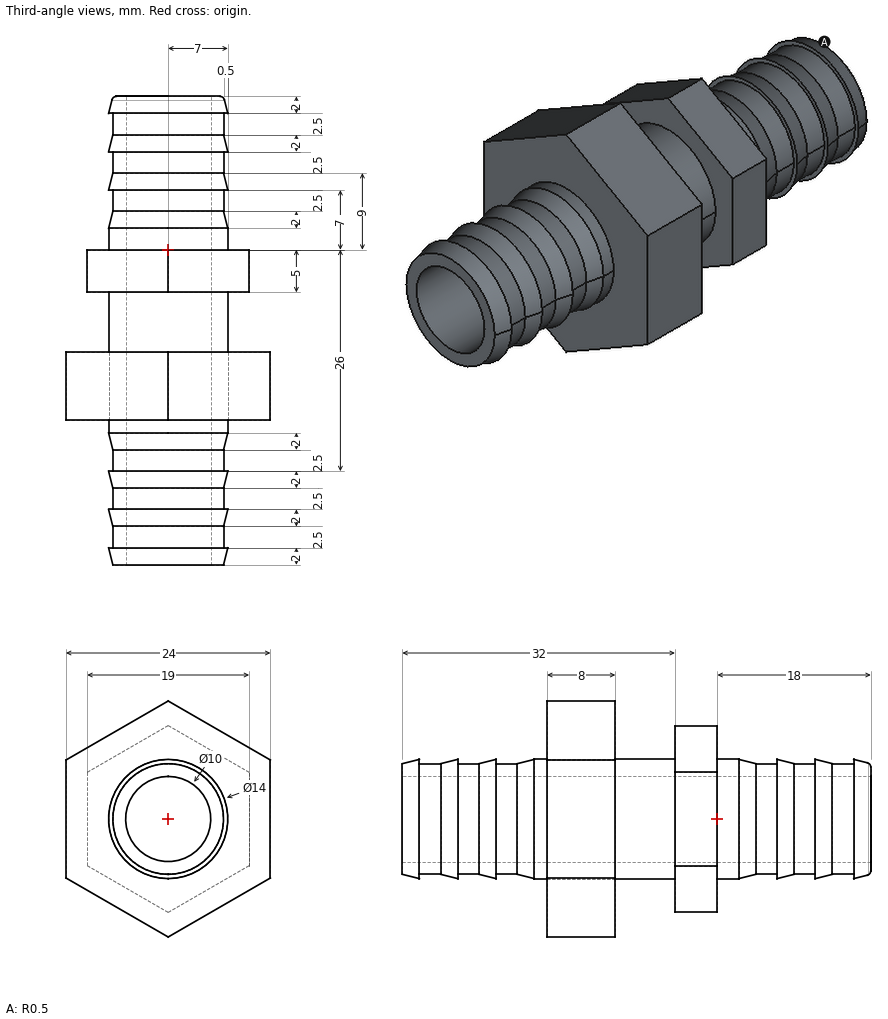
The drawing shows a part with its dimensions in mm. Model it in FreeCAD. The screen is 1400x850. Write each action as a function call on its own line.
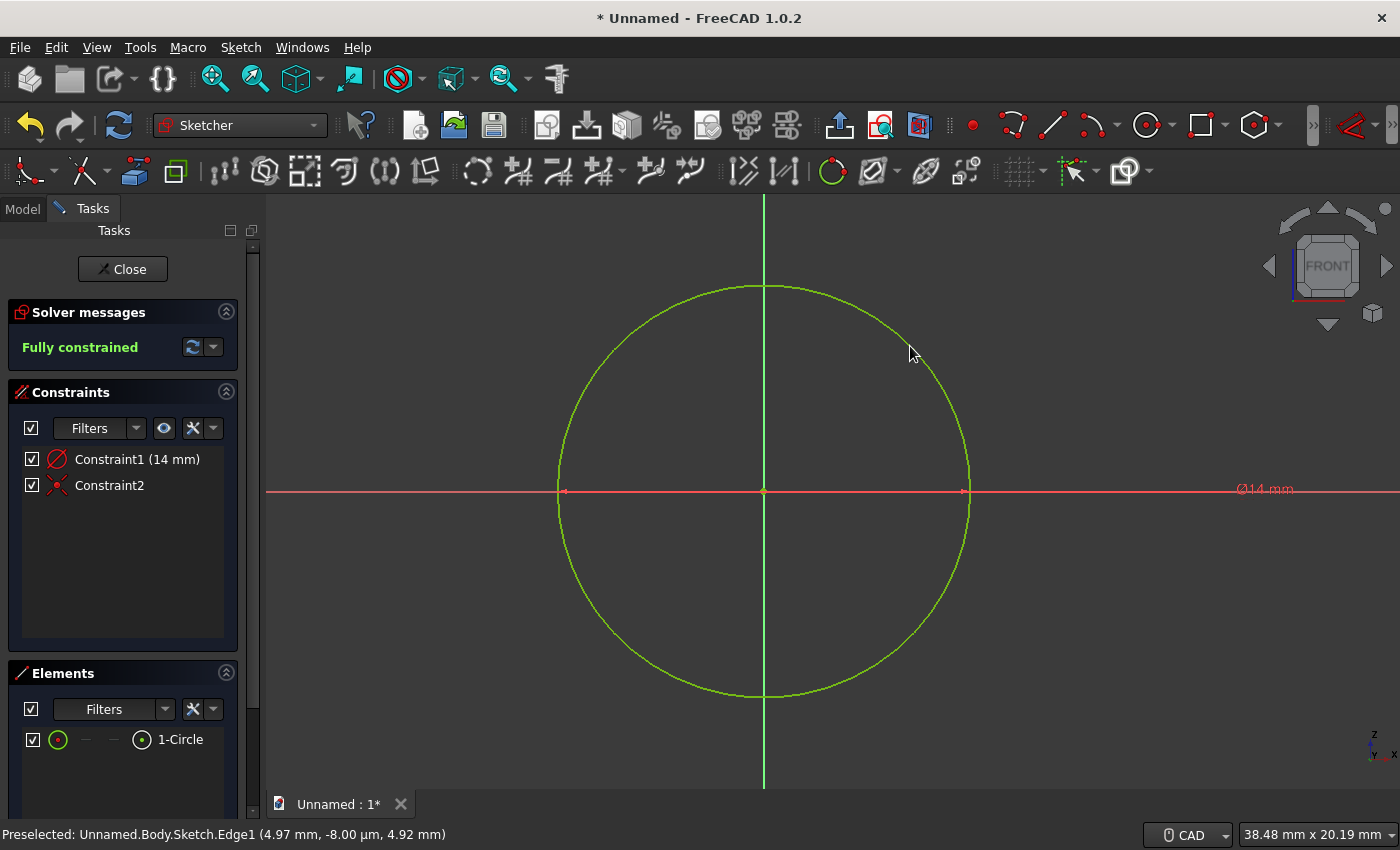
click(123, 269)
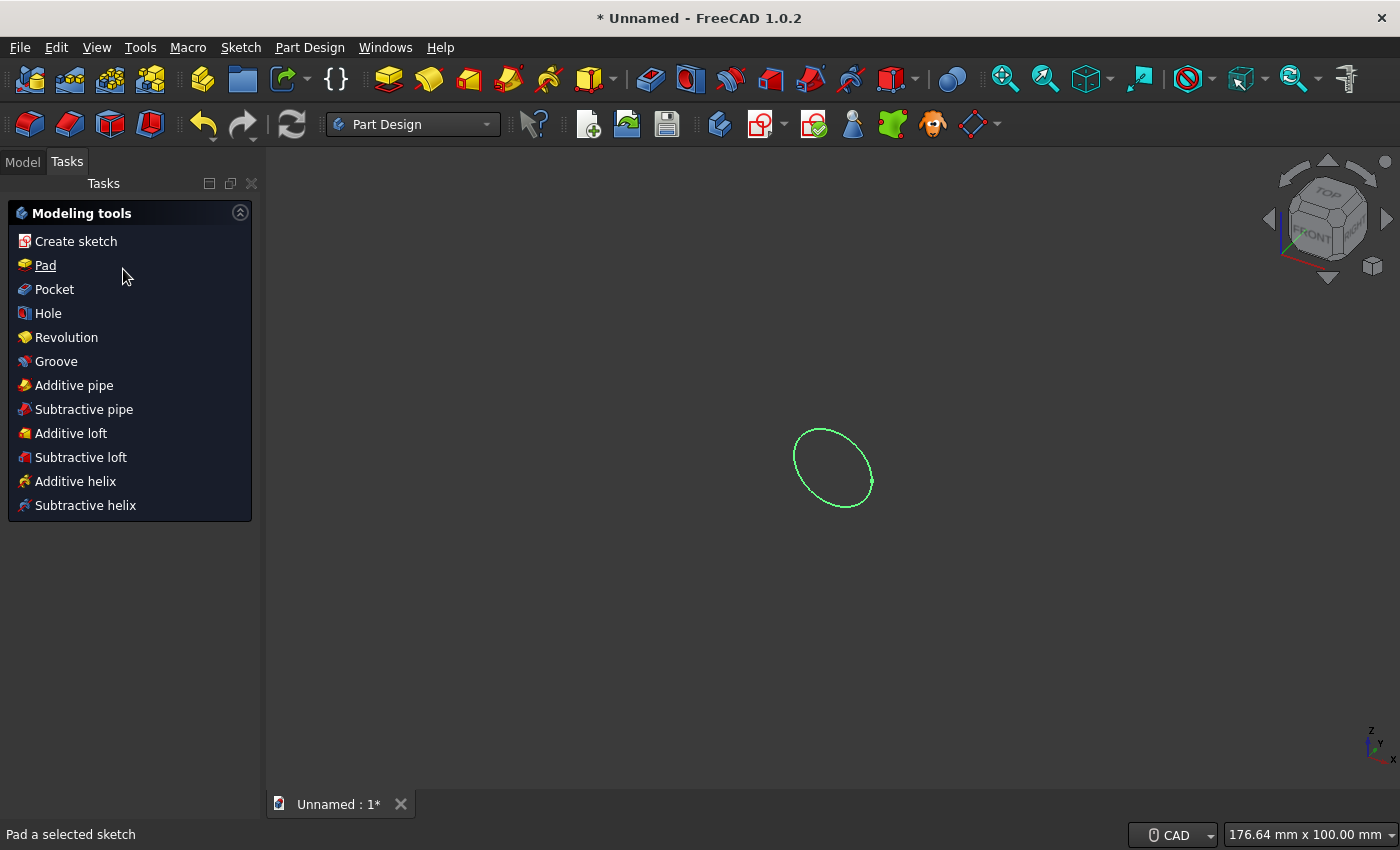
click(390, 80)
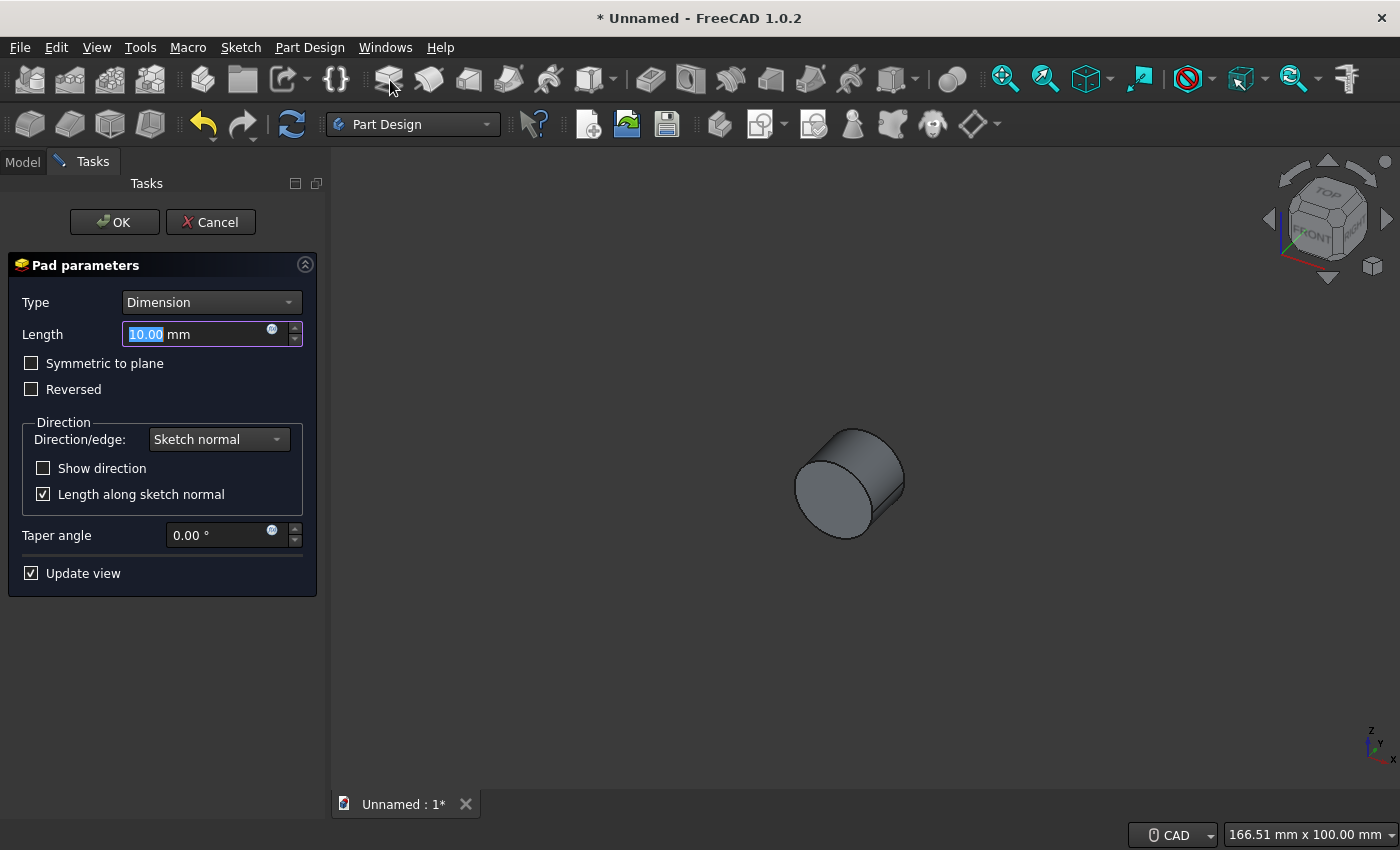
text(18)
key(Tab)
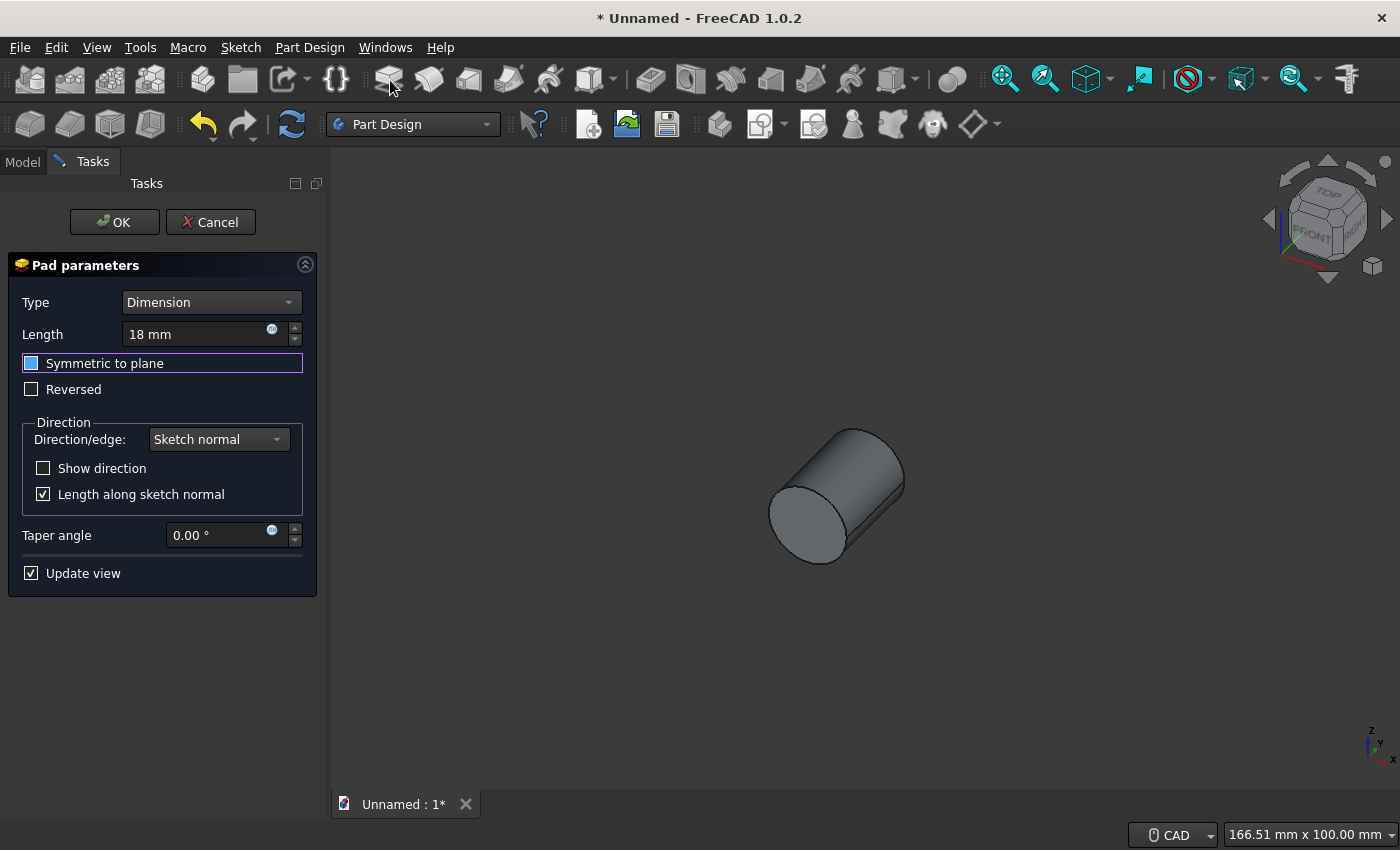
click(30, 389)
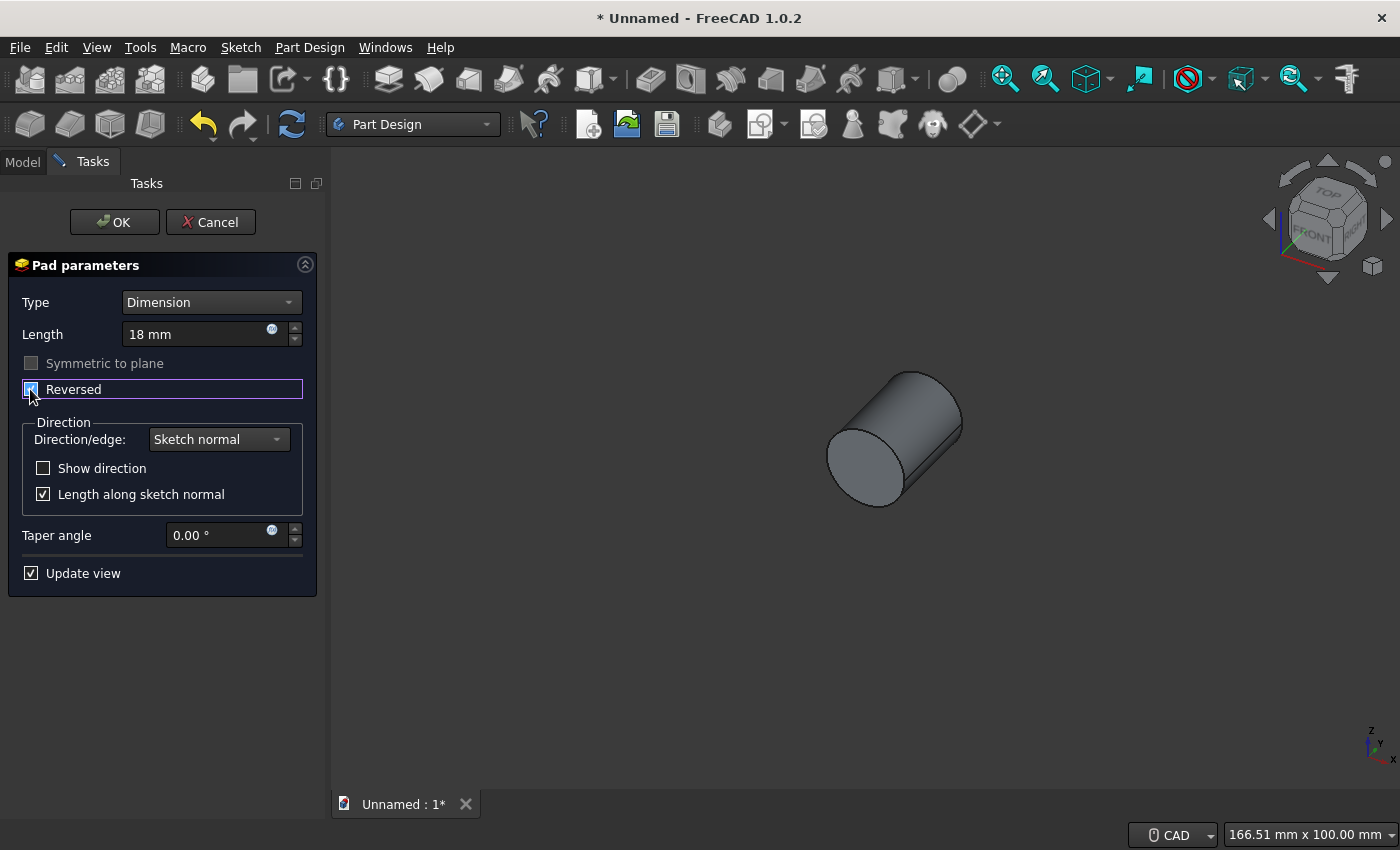
click(115, 222)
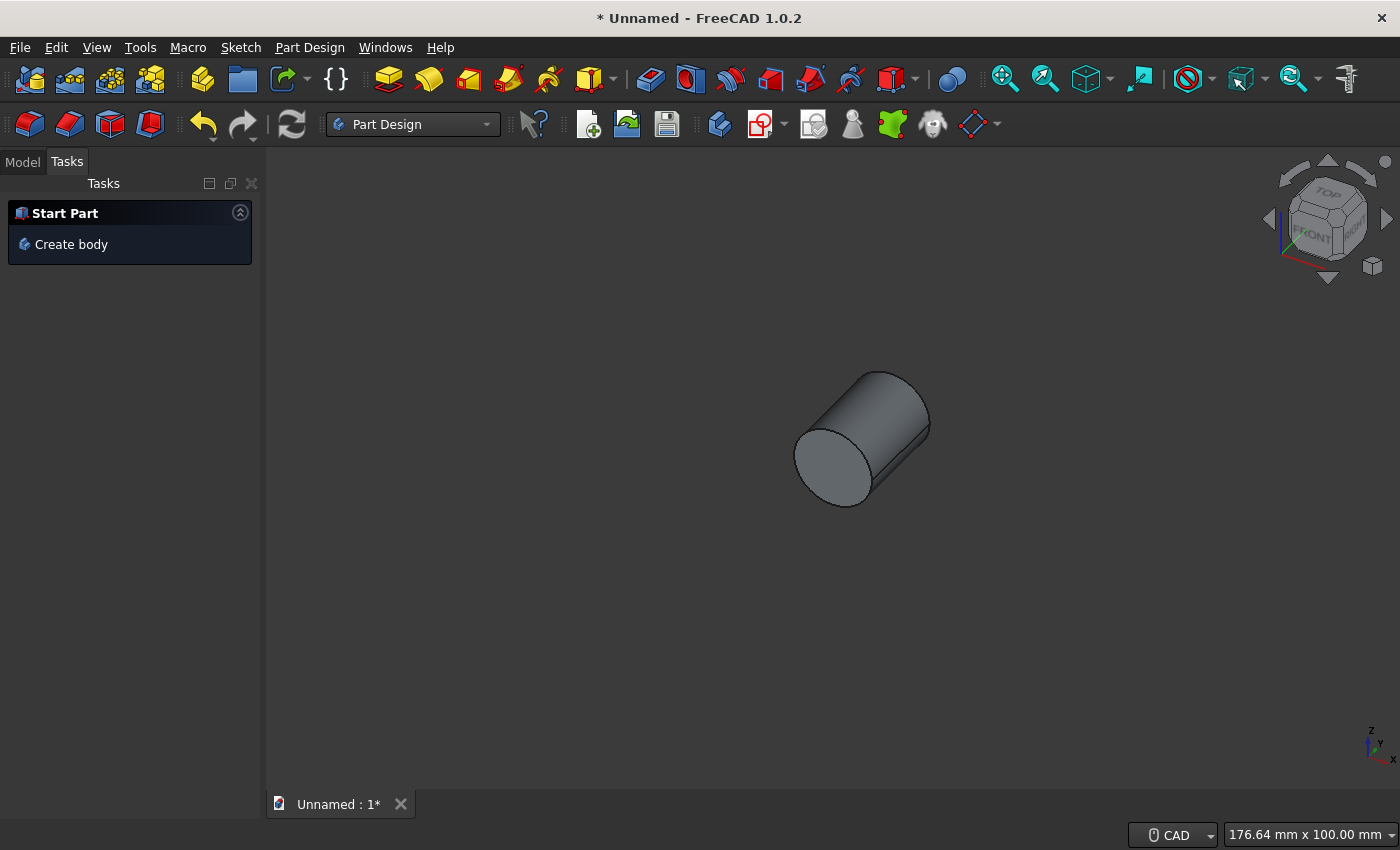
click(1006, 80)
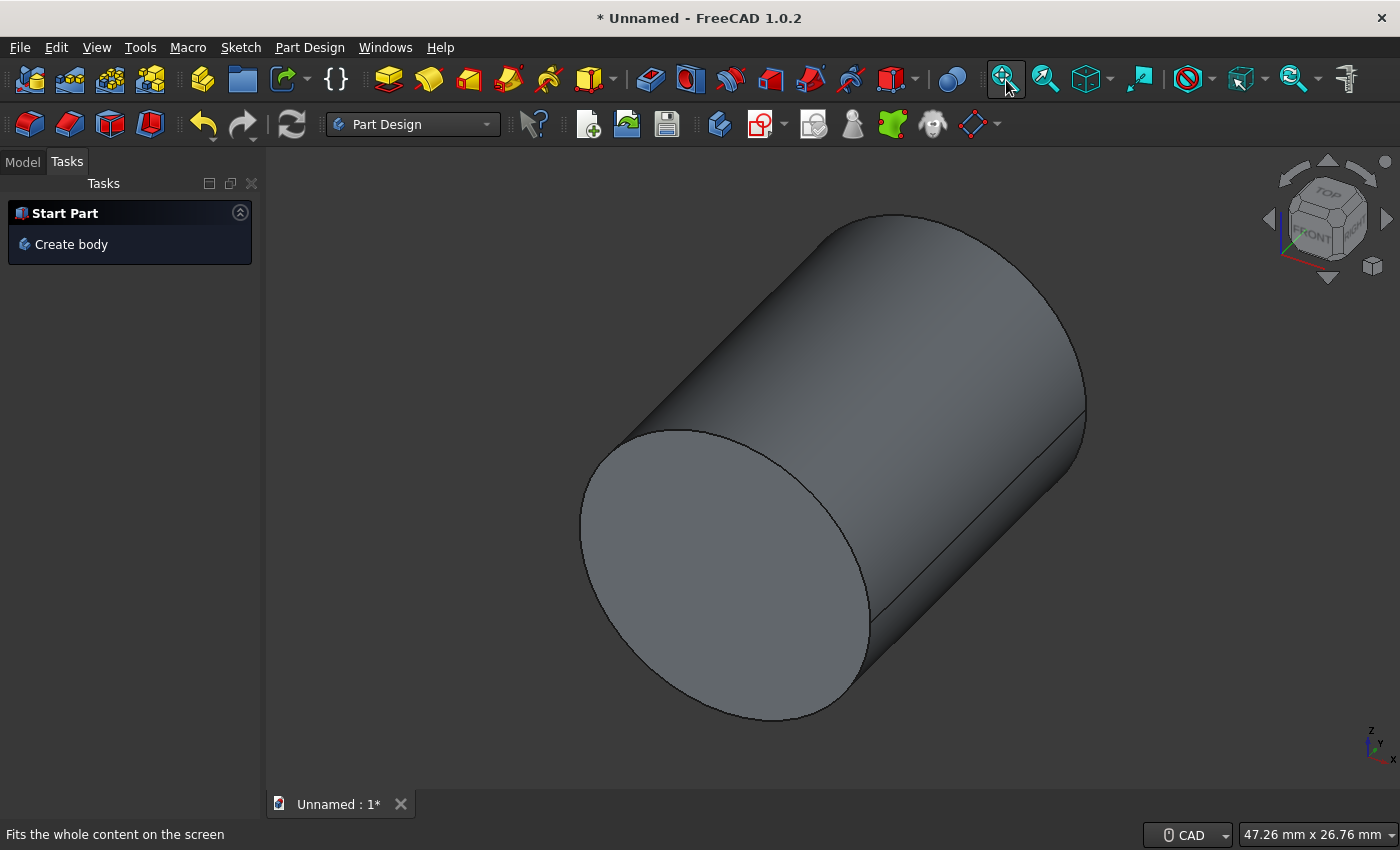
click(725, 574)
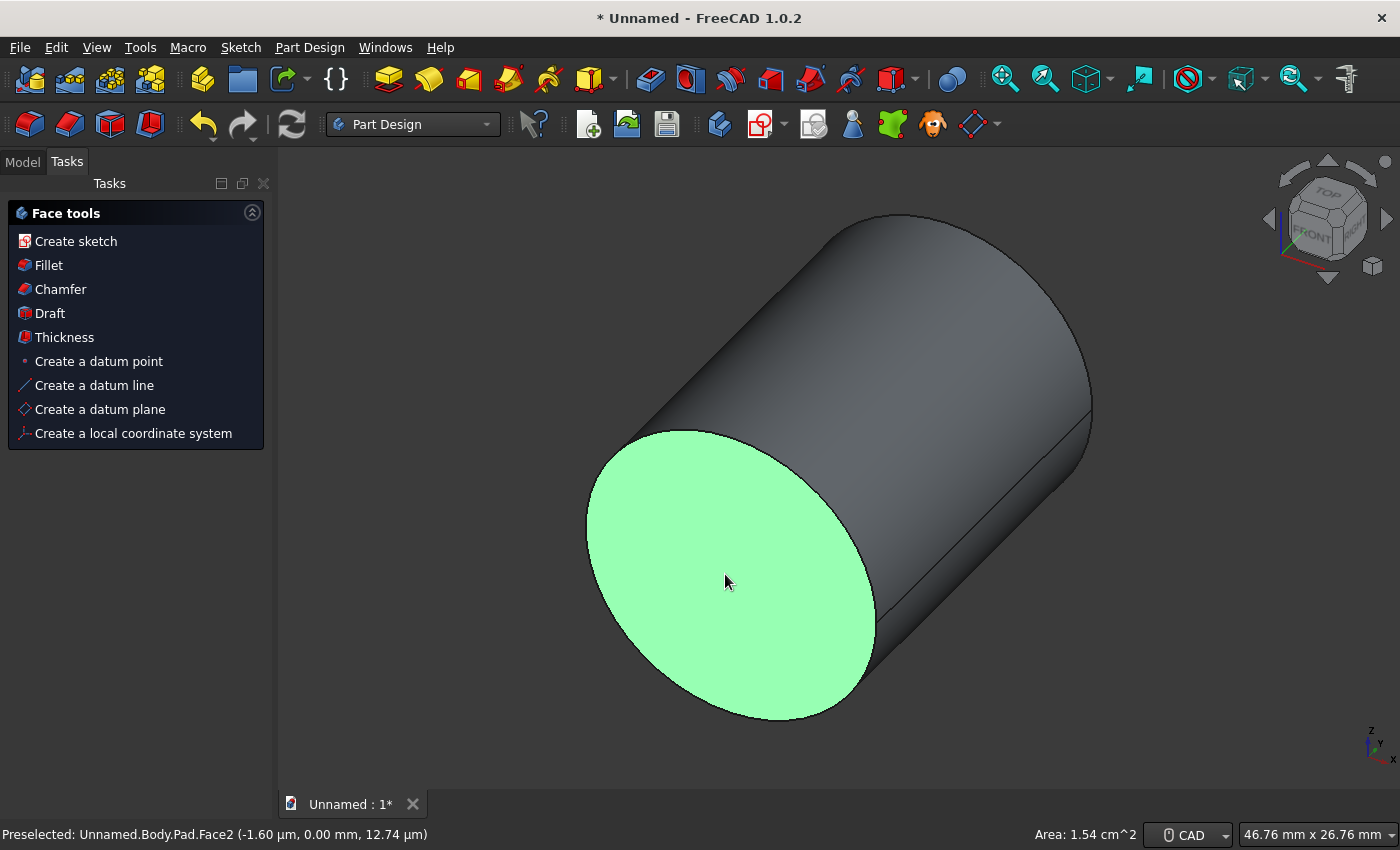
click(760, 124)